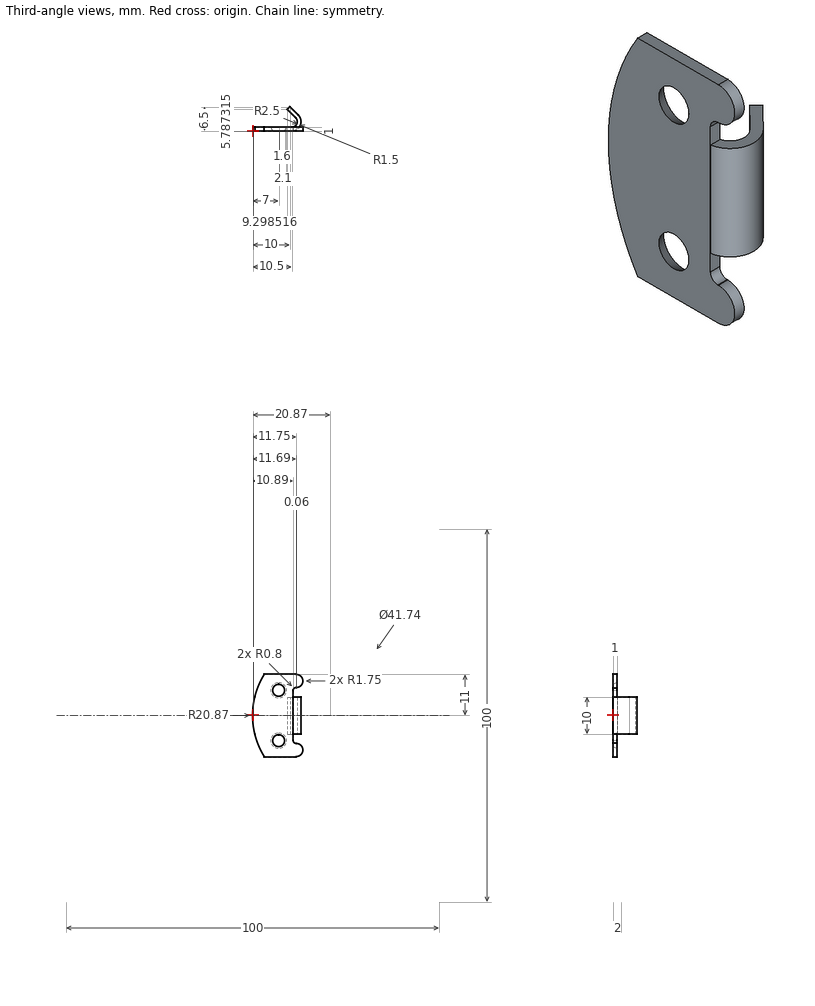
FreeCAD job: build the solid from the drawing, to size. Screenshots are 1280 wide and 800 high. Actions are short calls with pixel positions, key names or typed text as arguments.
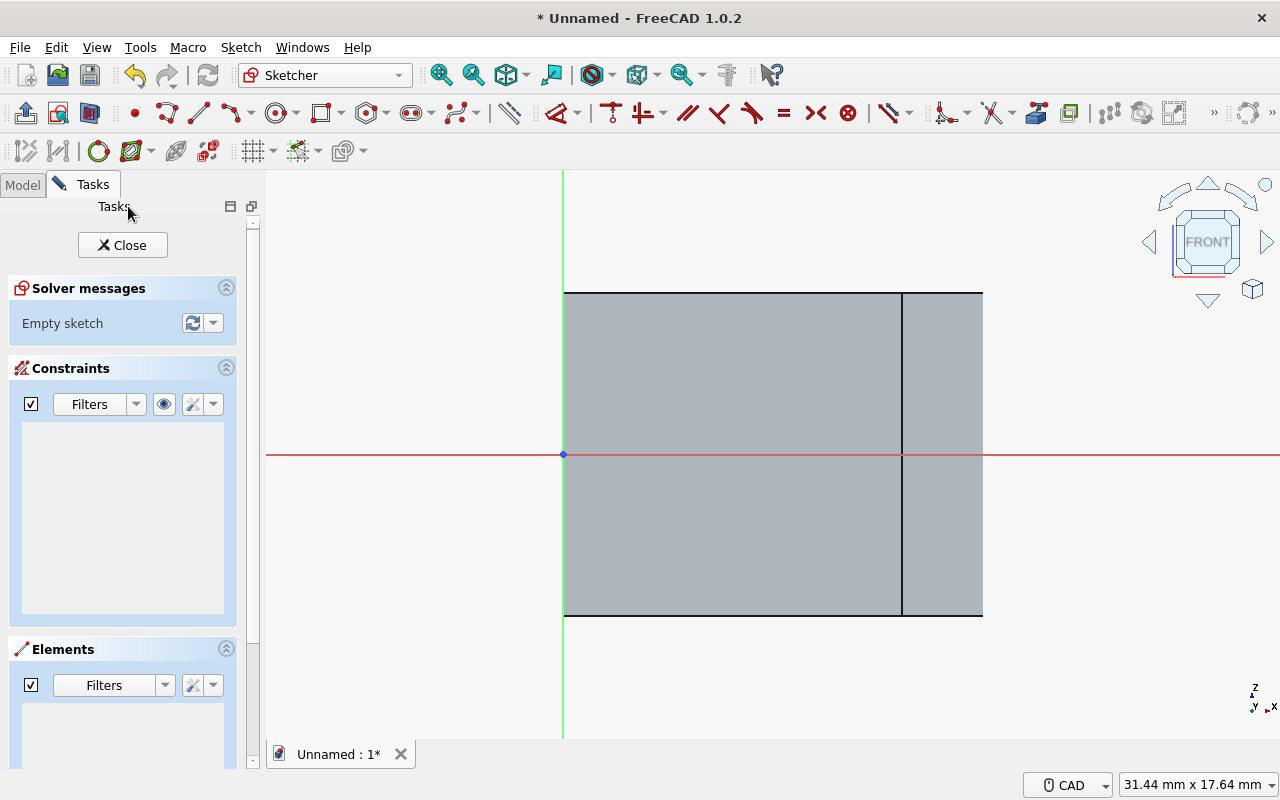
scroll(611, 454, down, 3)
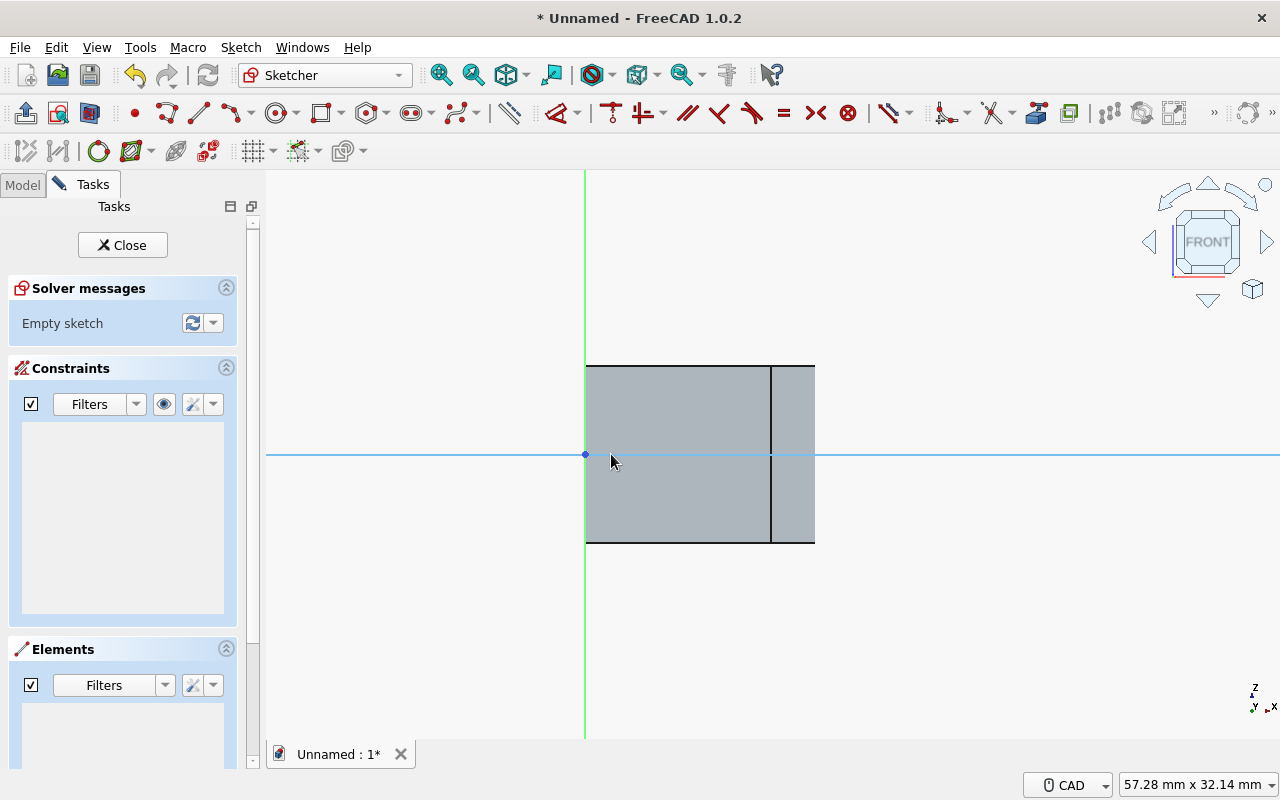
click(200, 114)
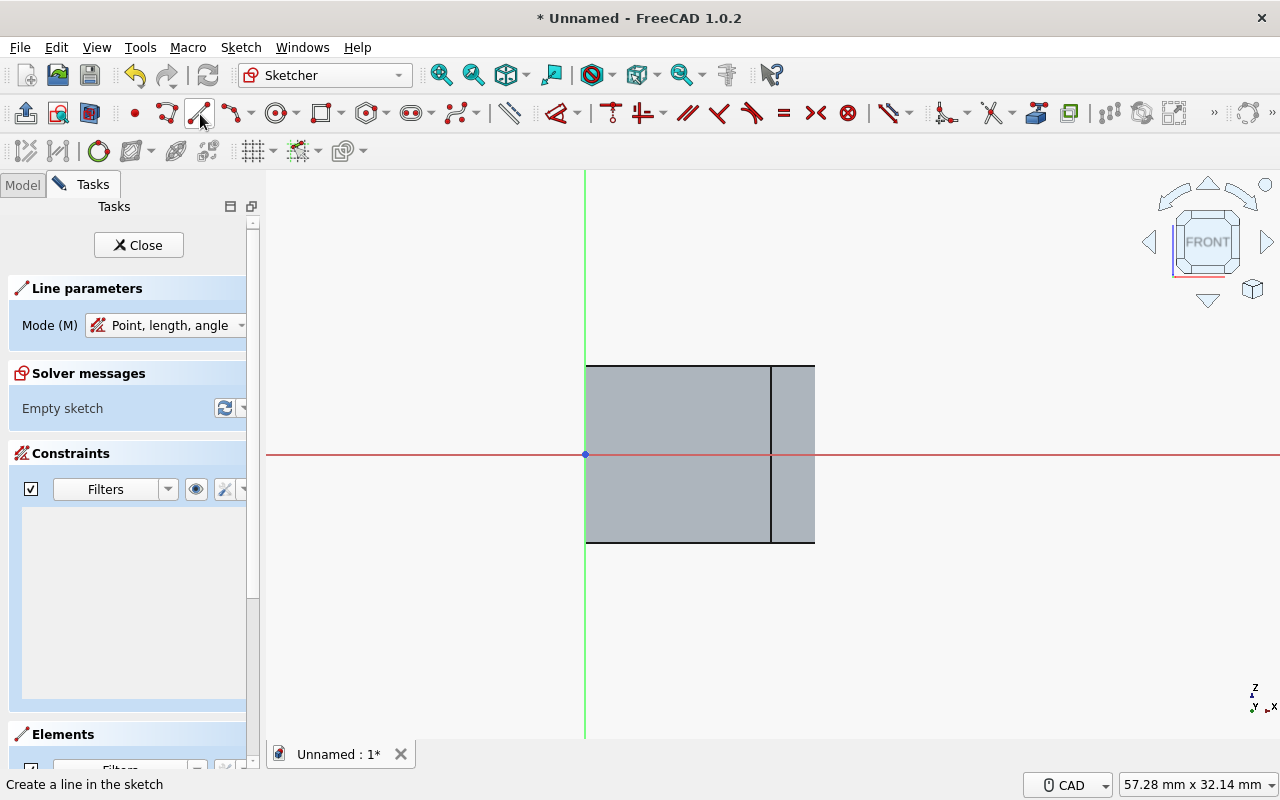
click(641, 260)
click(793, 260)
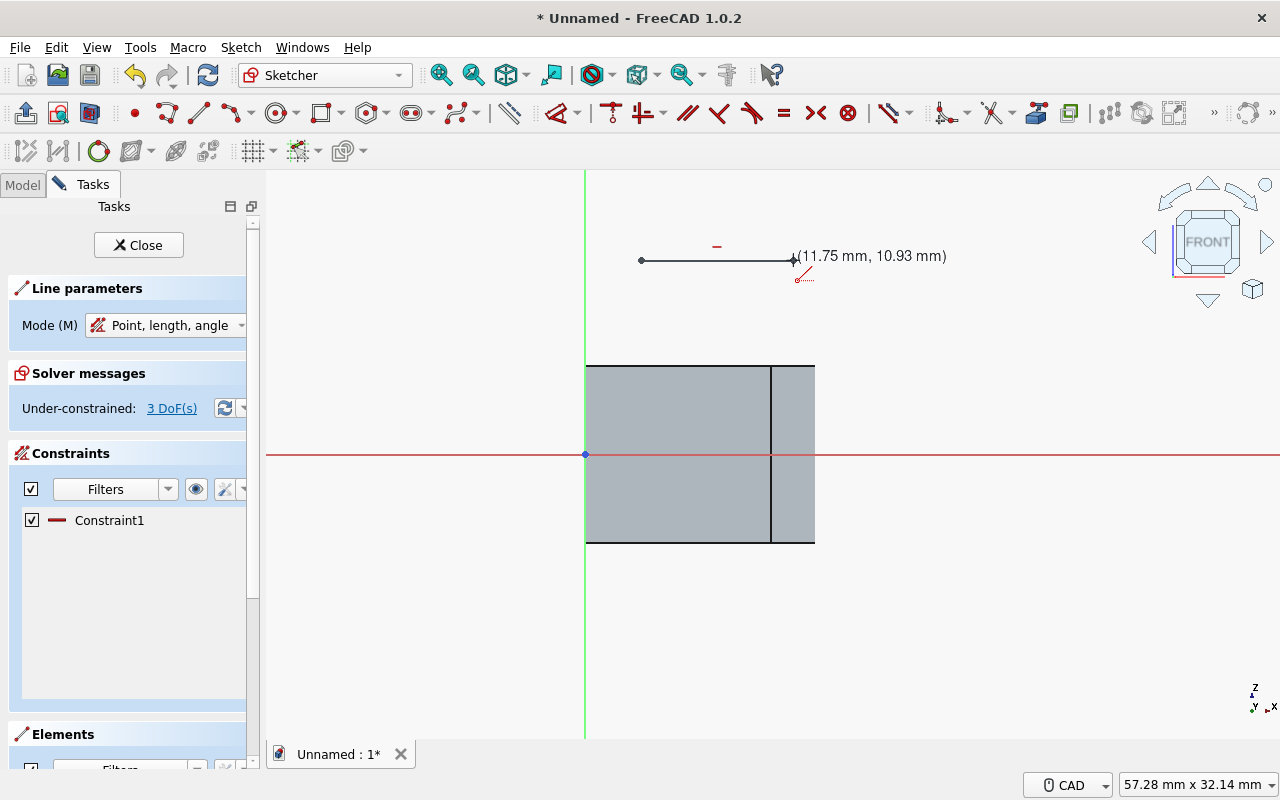
click(793, 322)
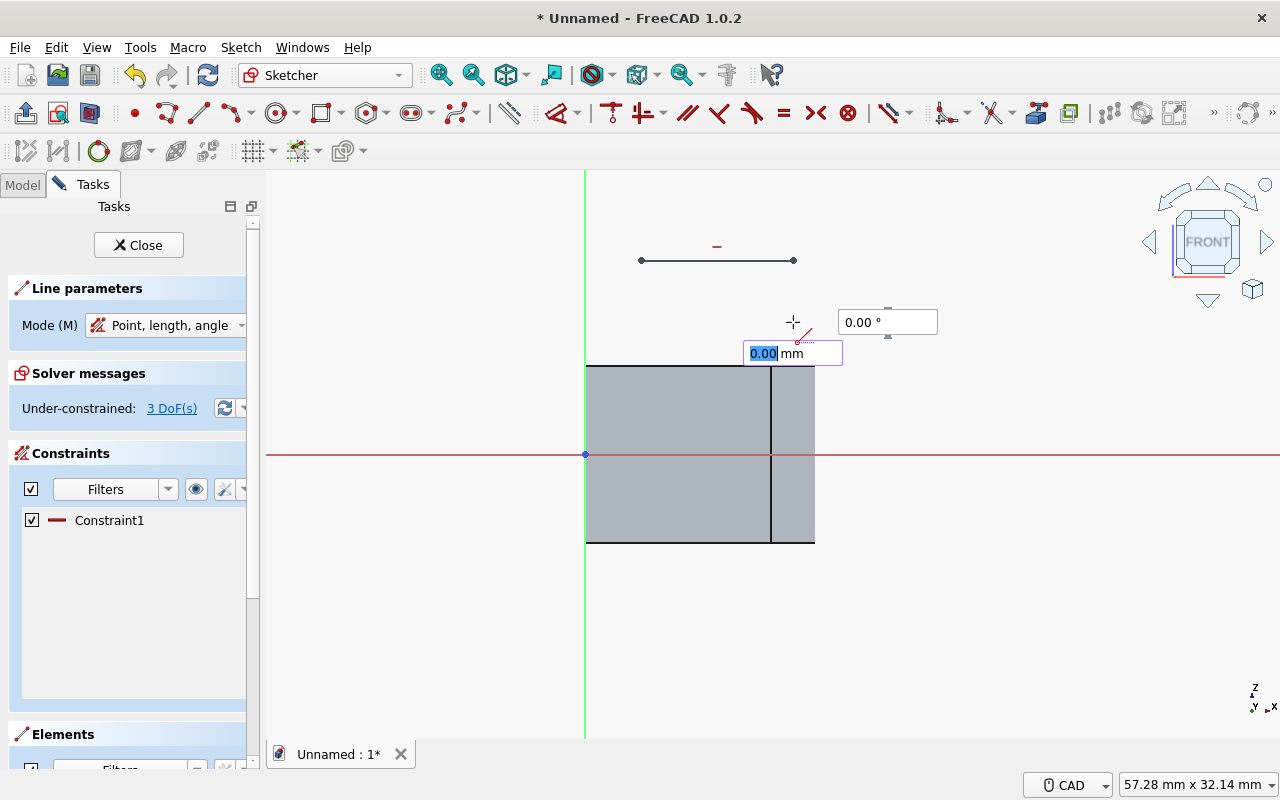
scroll(792, 322, up, 14)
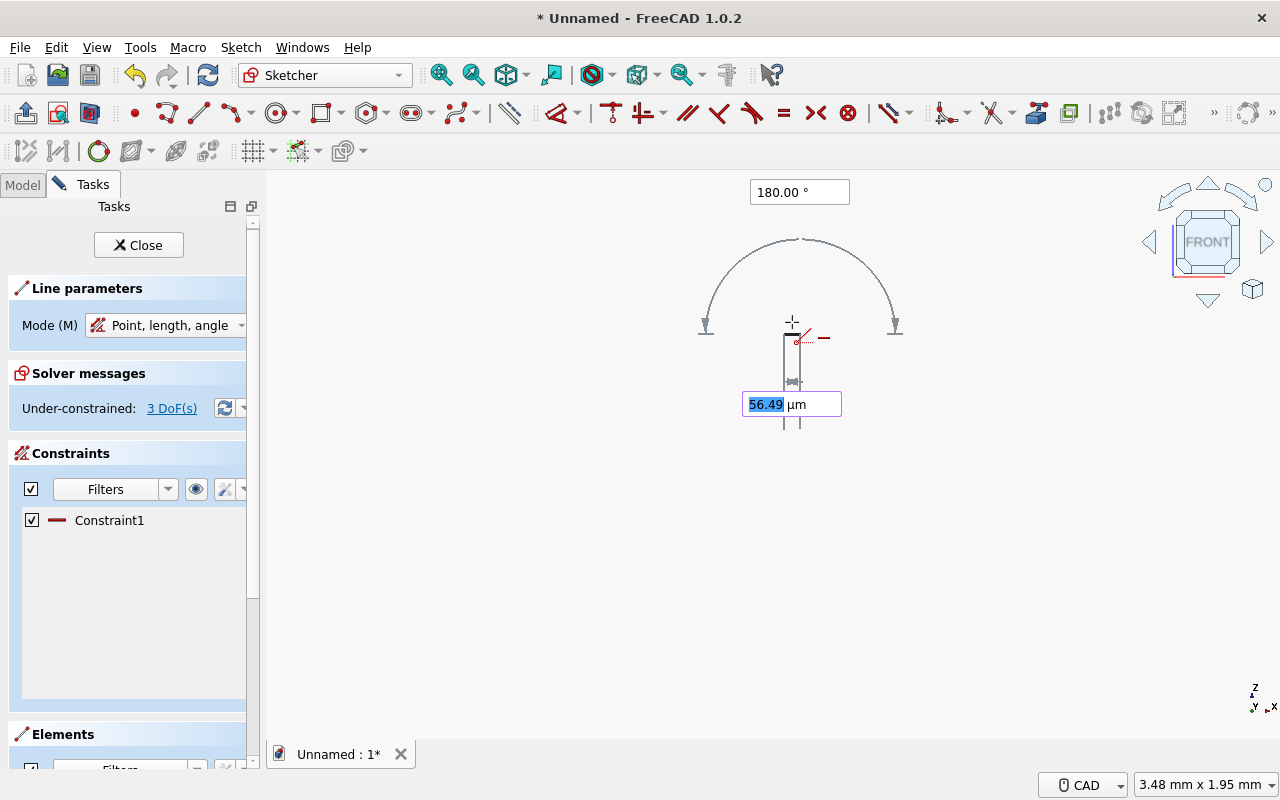
click(783, 318)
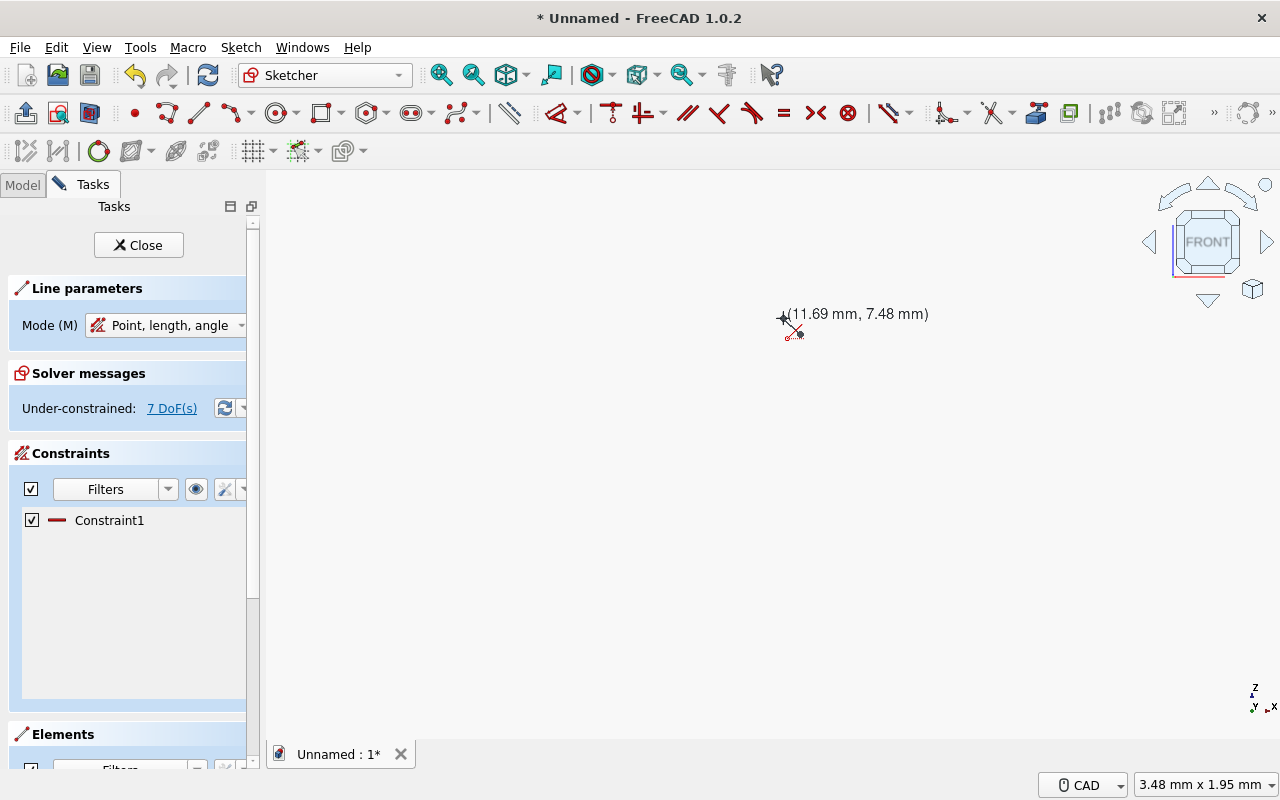
scroll(793, 322, down, 14)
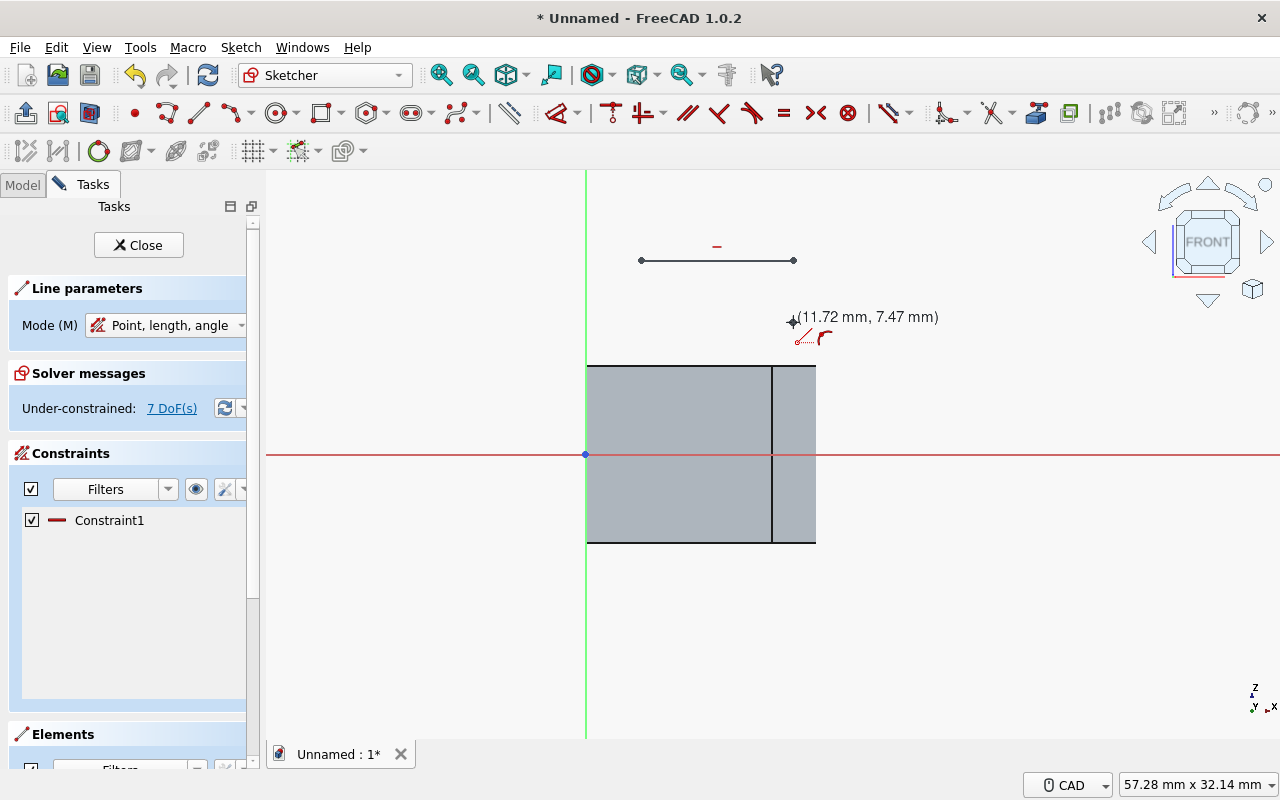
click(779, 336)
click(779, 573)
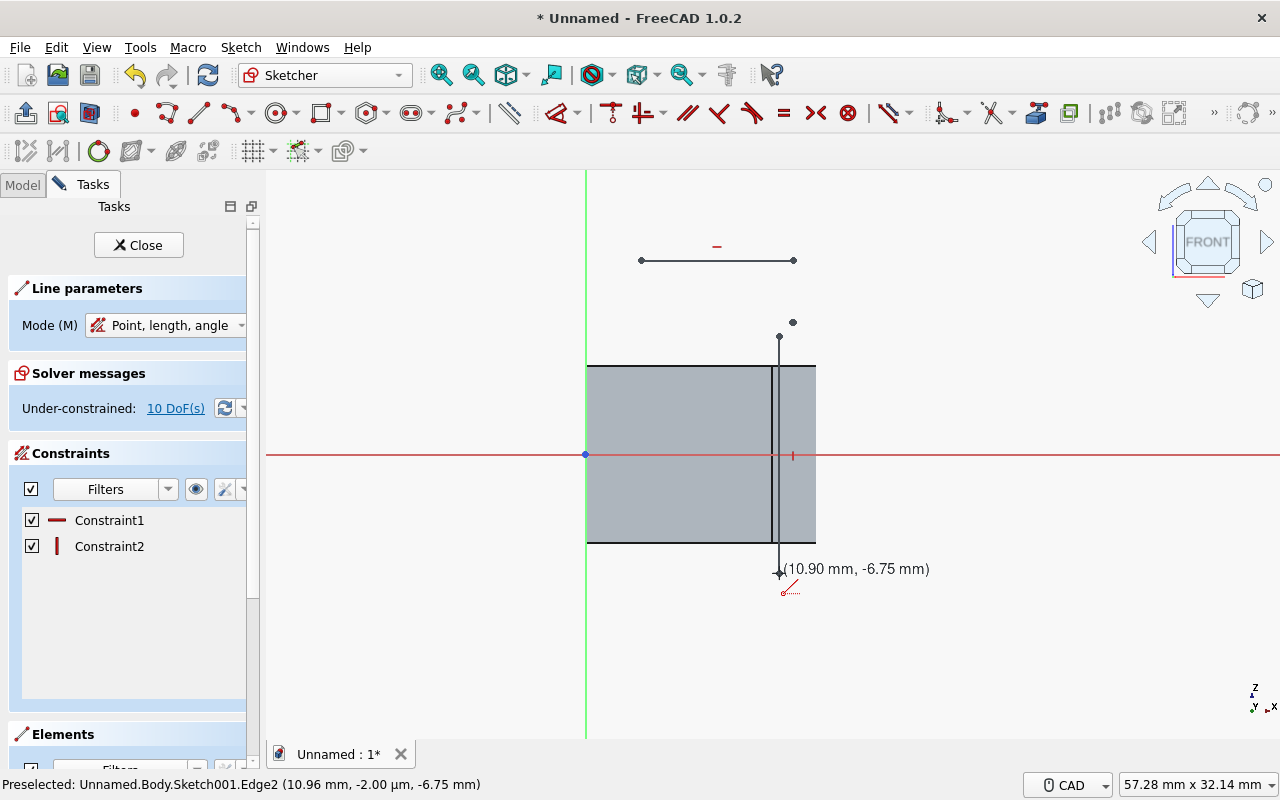
click(793, 587)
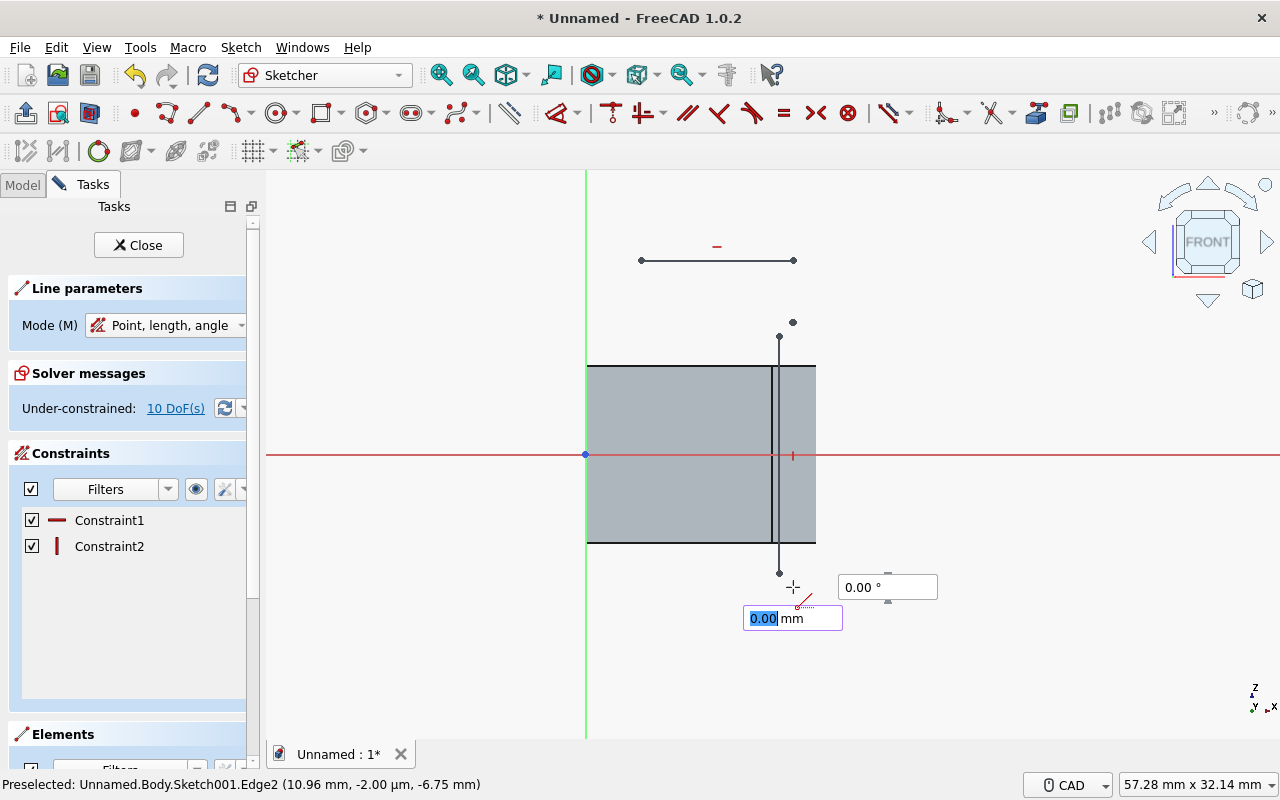
scroll(794, 587, up, 14)